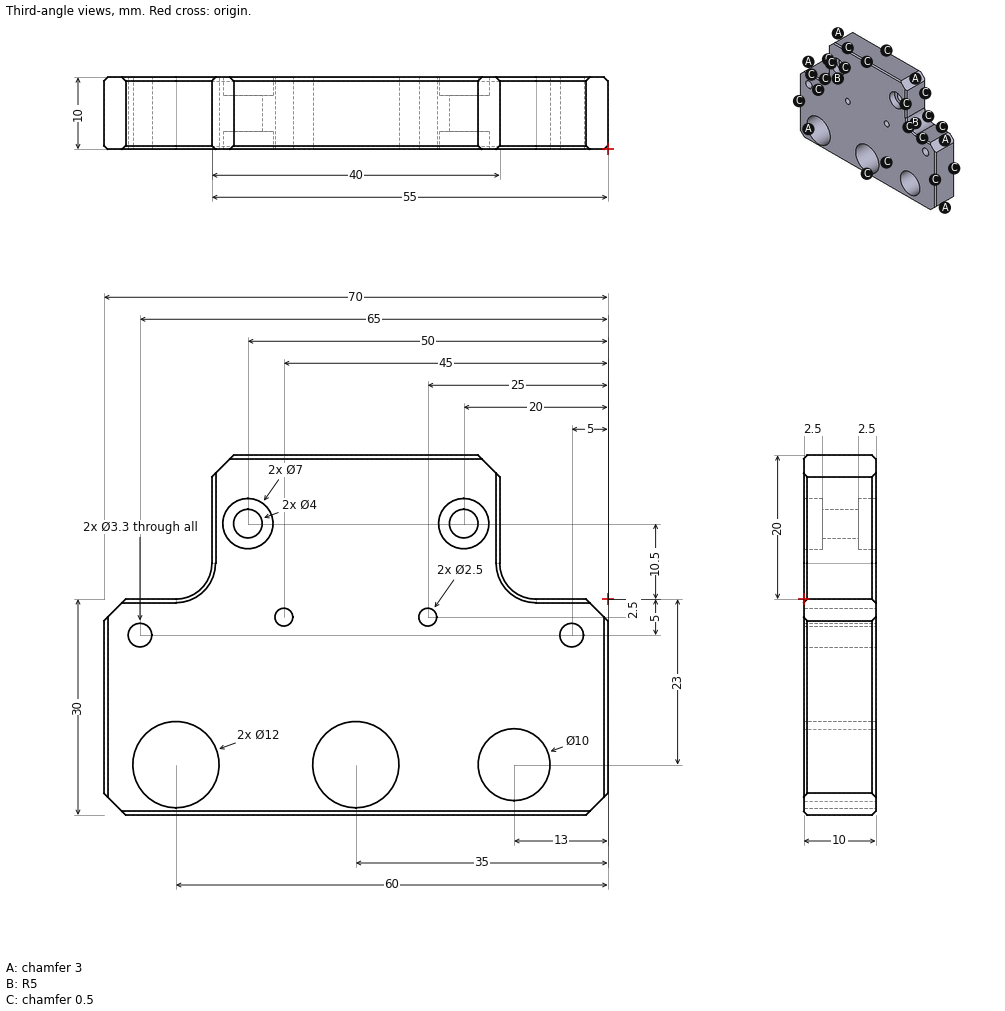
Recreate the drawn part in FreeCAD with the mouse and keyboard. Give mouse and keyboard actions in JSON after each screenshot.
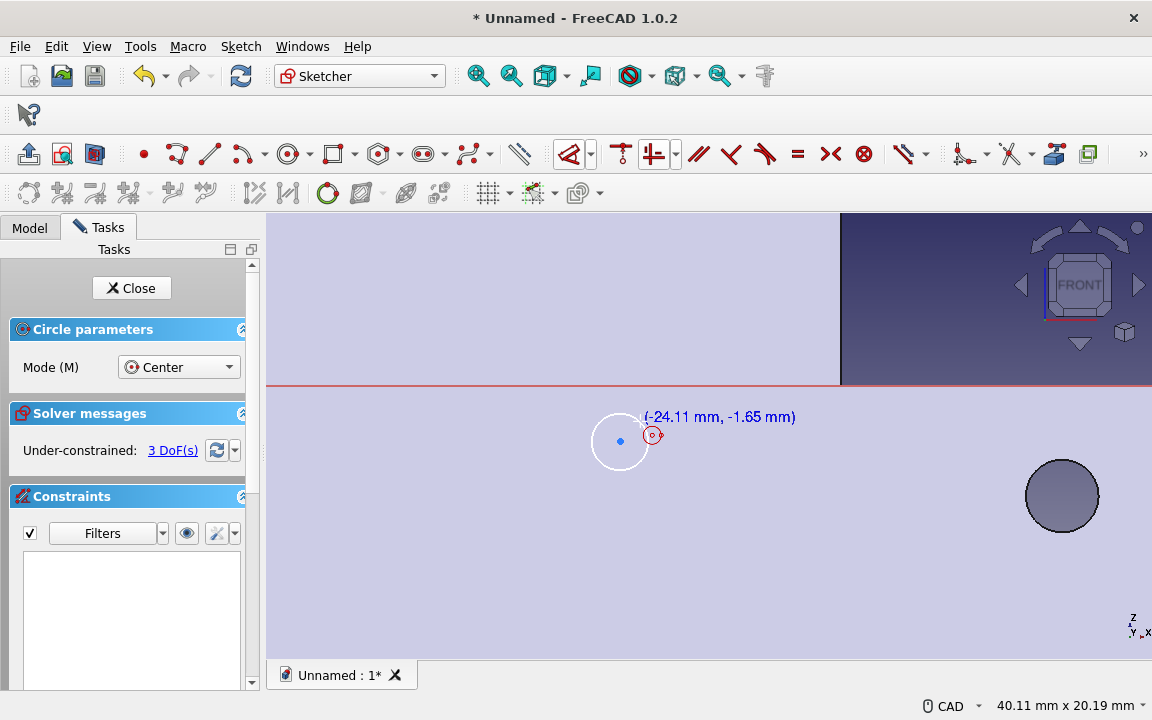
{"action": "scroll", "coordinate": [623, 443], "scroll_direction": "down", "scroll_amount": 4}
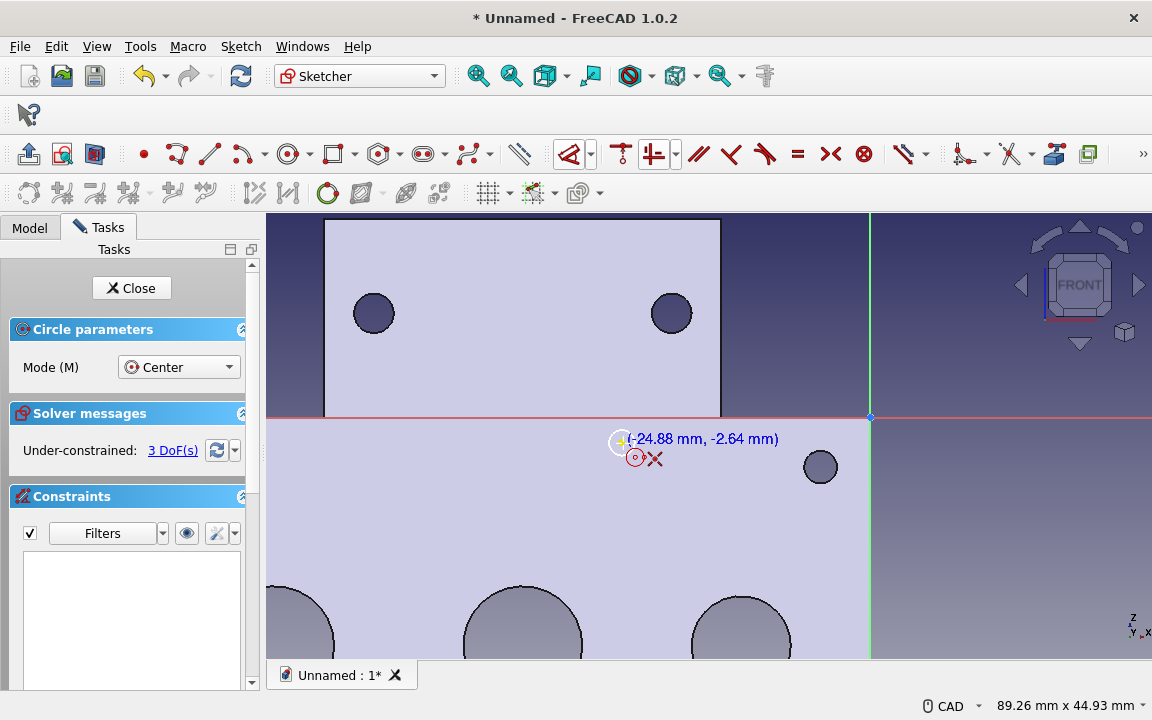
{"action": "scroll", "coordinate": [424, 442], "scroll_direction": "up", "scroll_amount": 4}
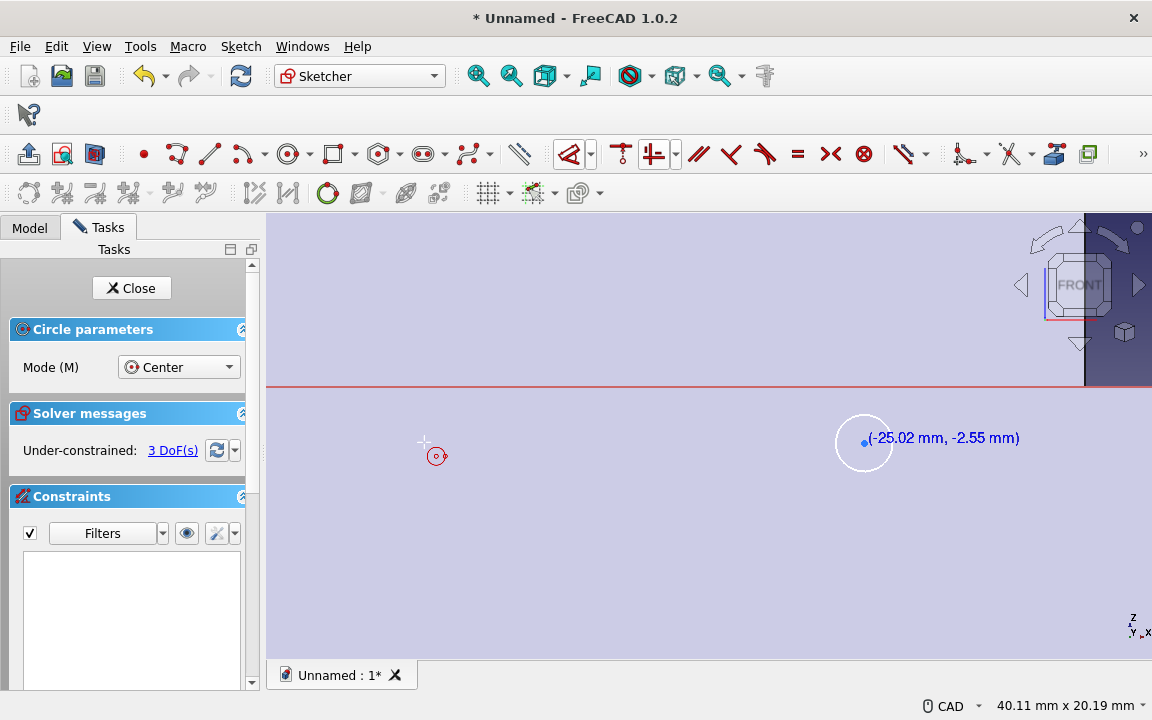
{"action": "left_click", "coordinate": [423, 442]}
{"action": "left_click", "coordinate": [442, 423]}
{"action": "key", "text": "Escape"}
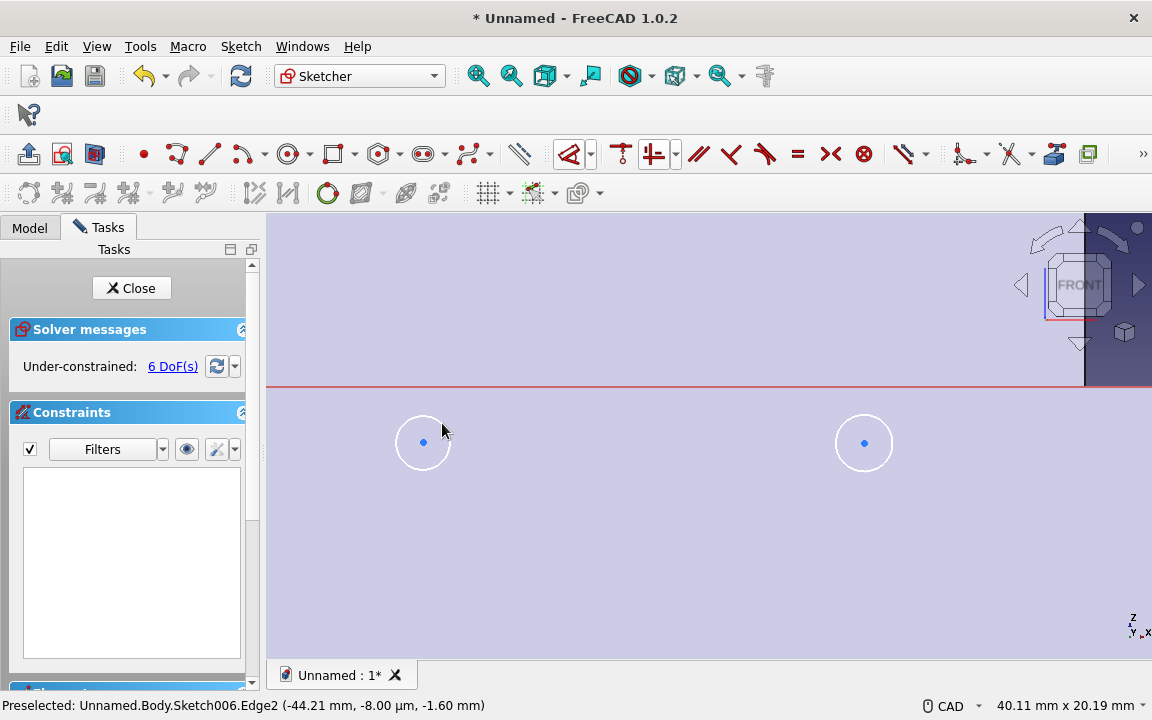
{"action": "left_click", "coordinate": [884, 423]}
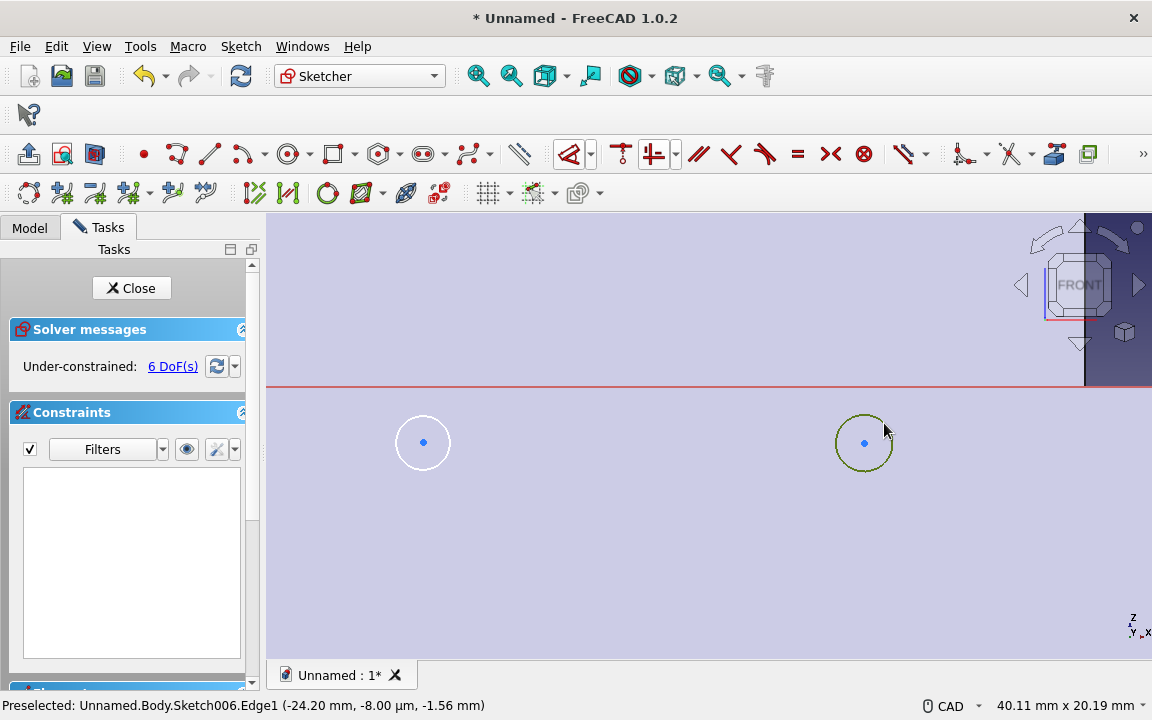
{"action": "left_click", "coordinate": [442, 424]}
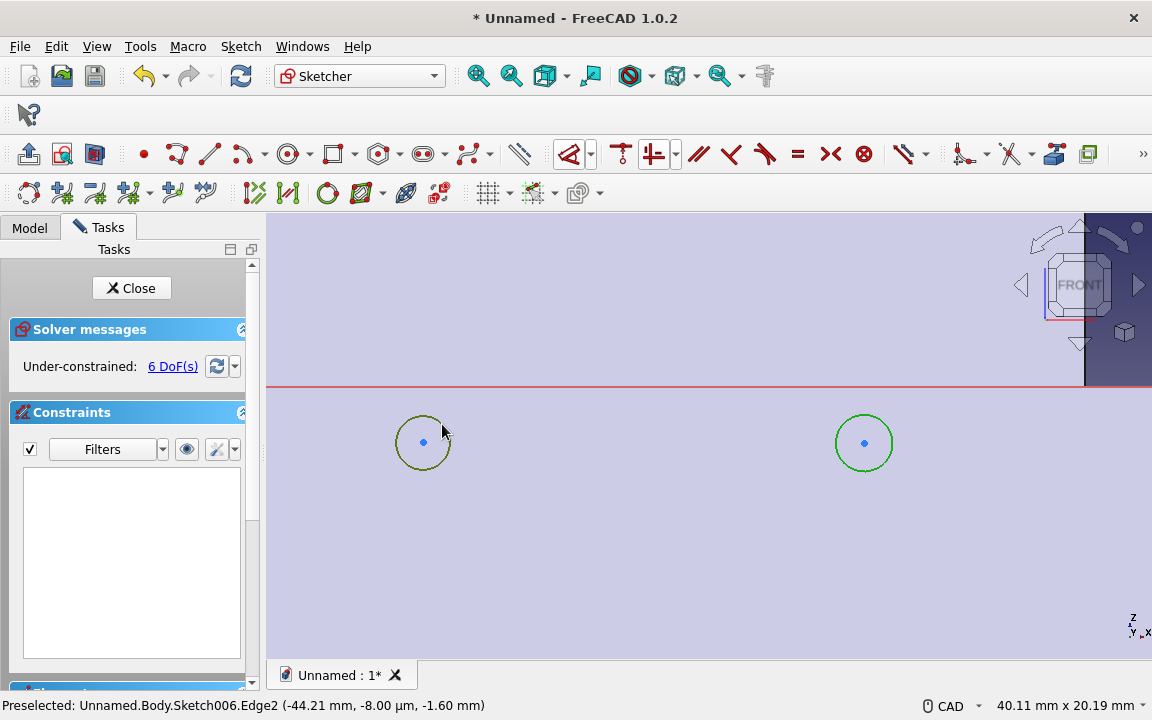
{"action": "left_click", "coordinate": [798, 154]}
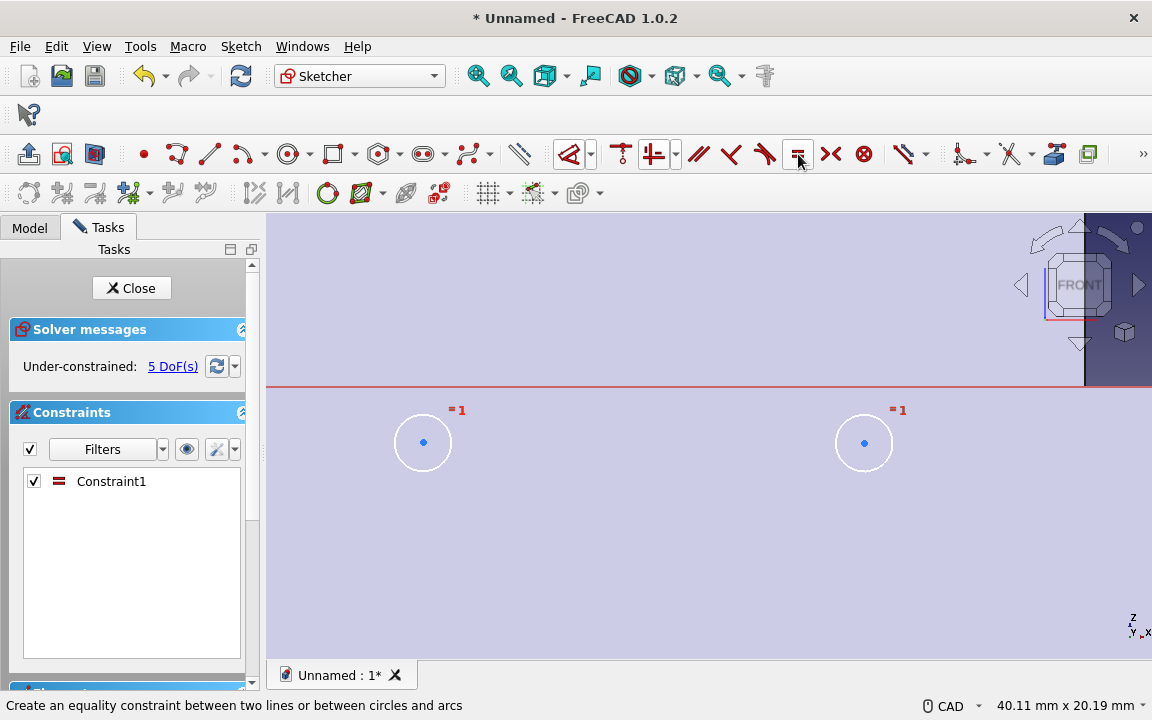
{"action": "left_click", "coordinate": [864, 443]}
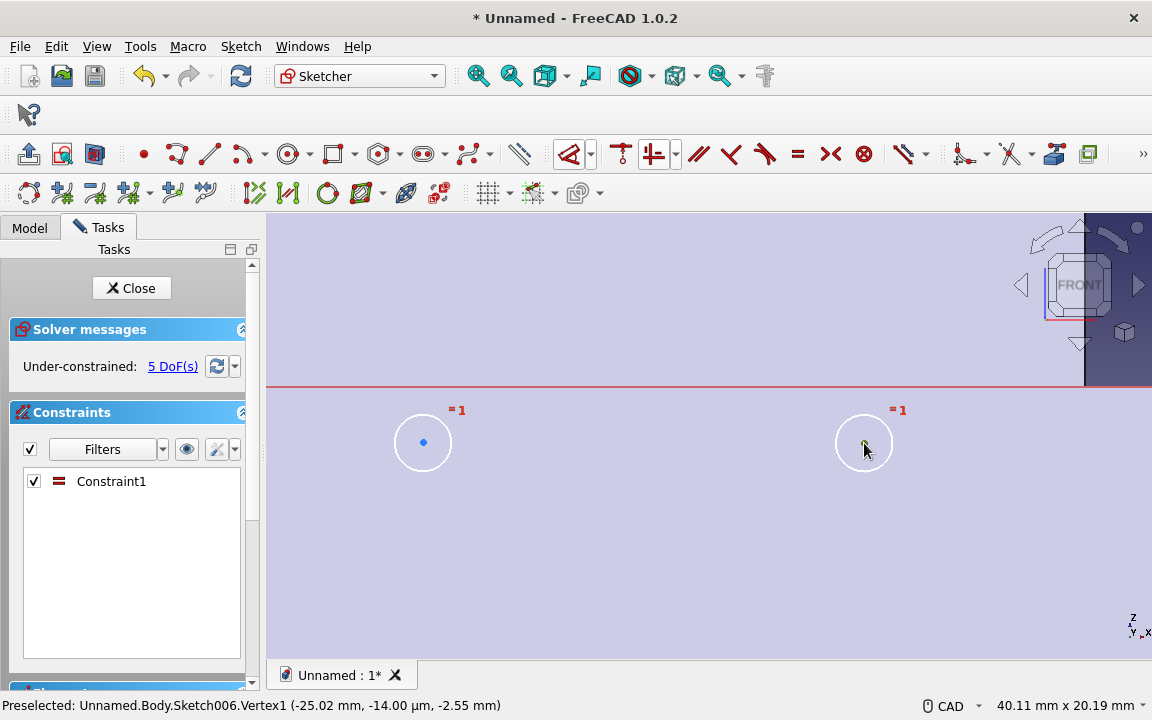
{"action": "left_click", "coordinate": [423, 443]}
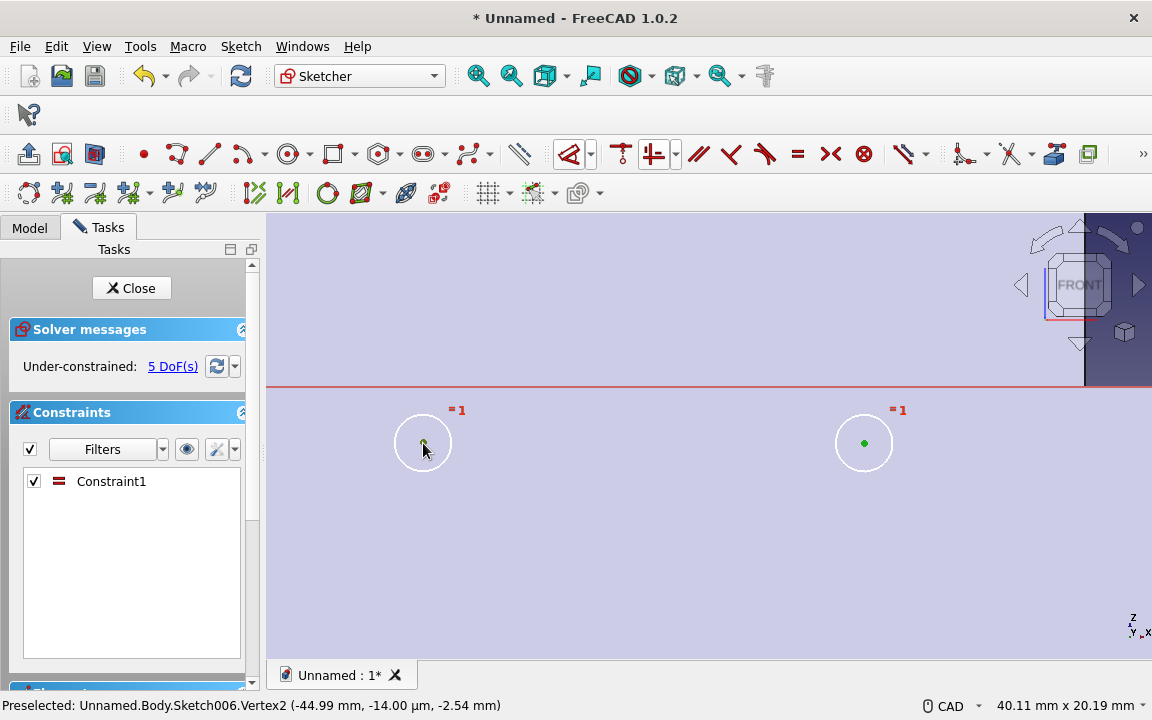
{"action": "left_click", "coordinate": [676, 154]}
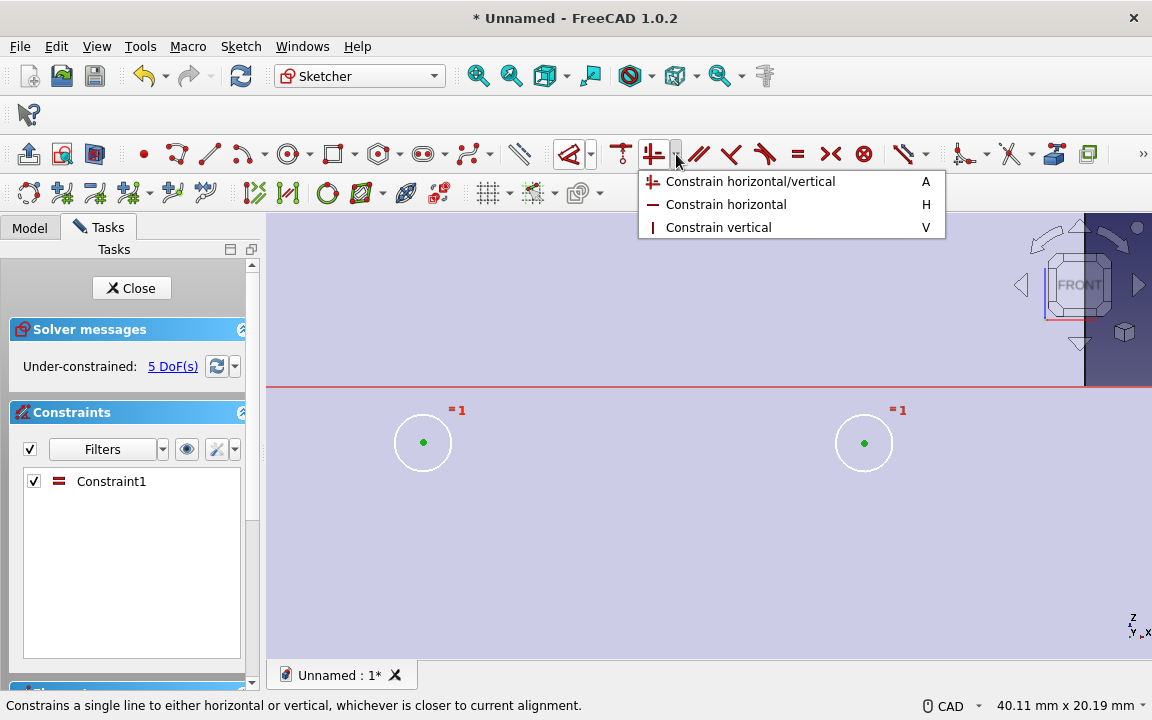
{"action": "left_click", "coordinate": [792, 204]}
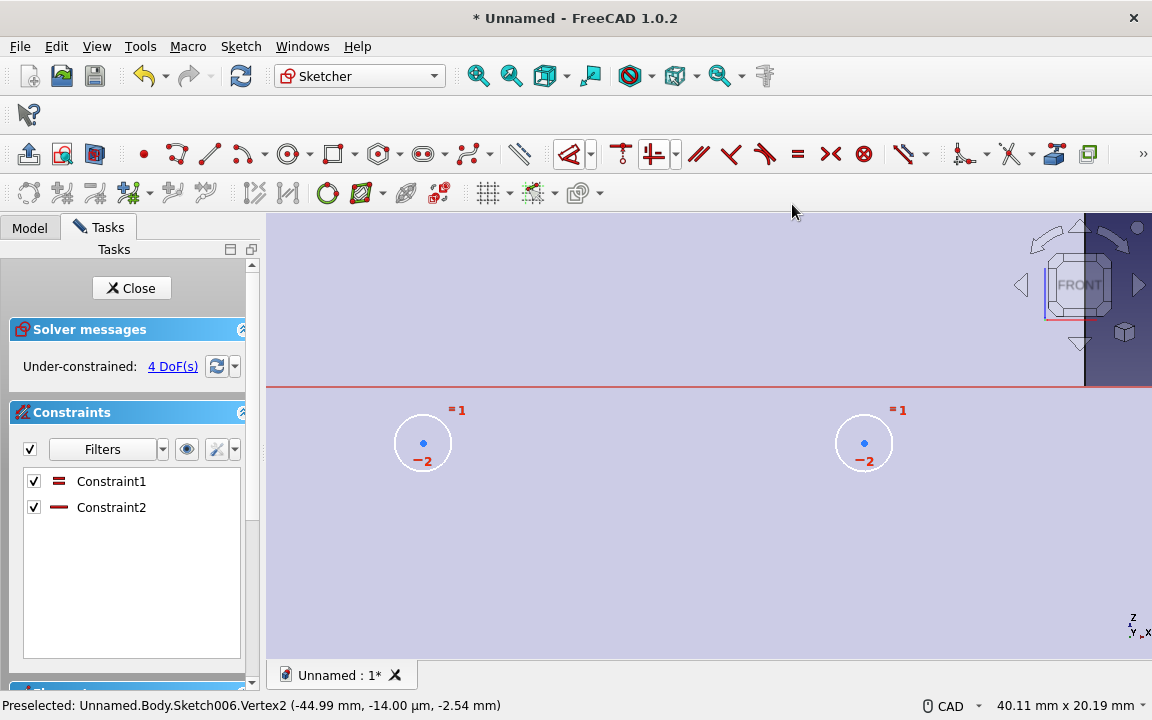
{"action": "left_click", "coordinate": [884, 423]}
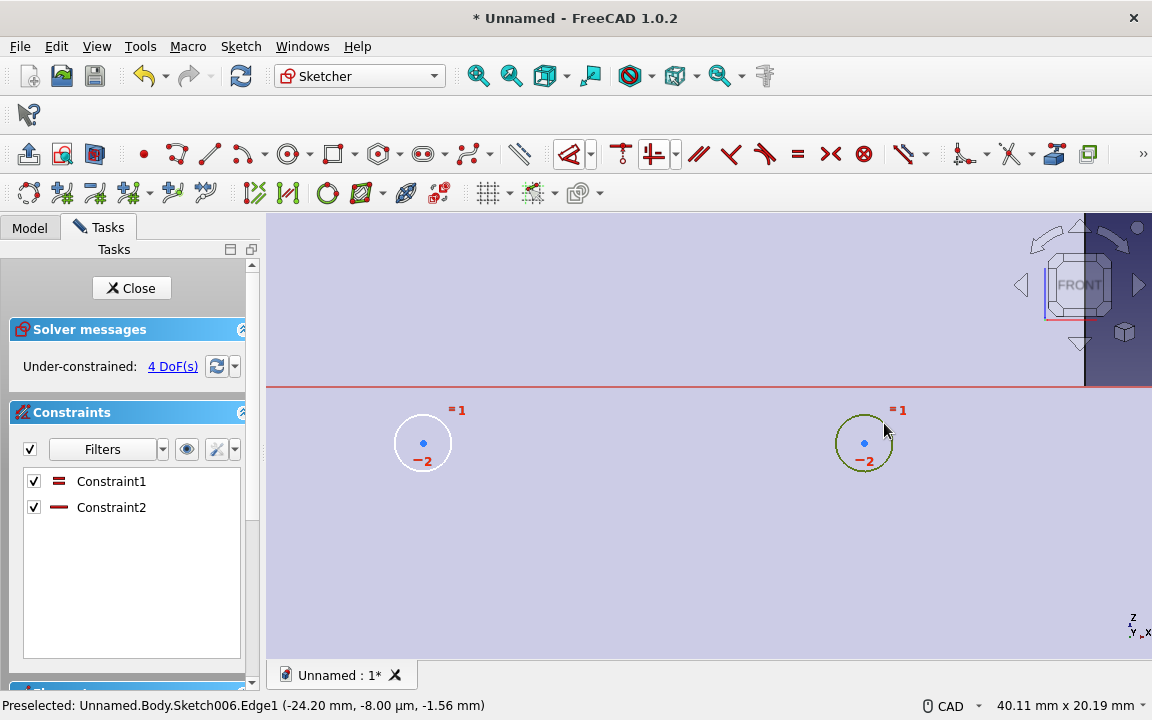
{"action": "key", "text": "k o"}